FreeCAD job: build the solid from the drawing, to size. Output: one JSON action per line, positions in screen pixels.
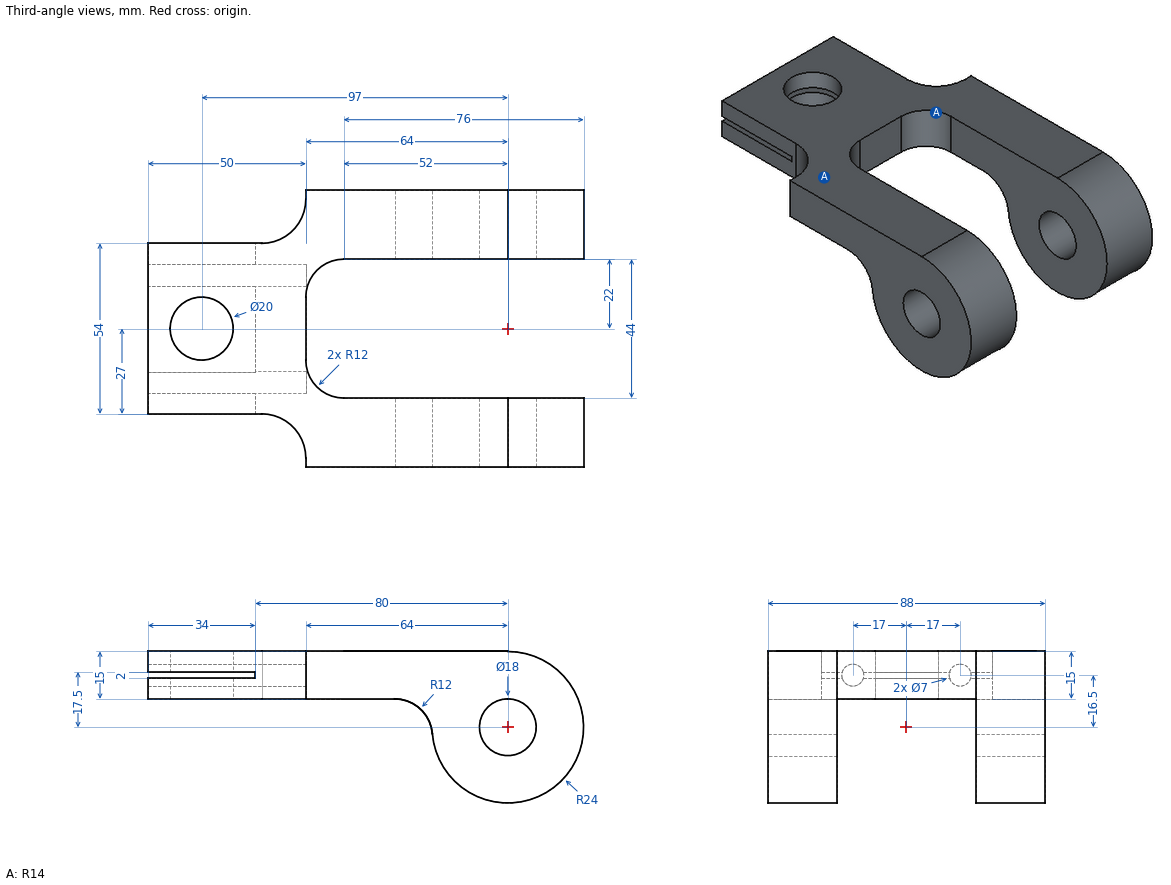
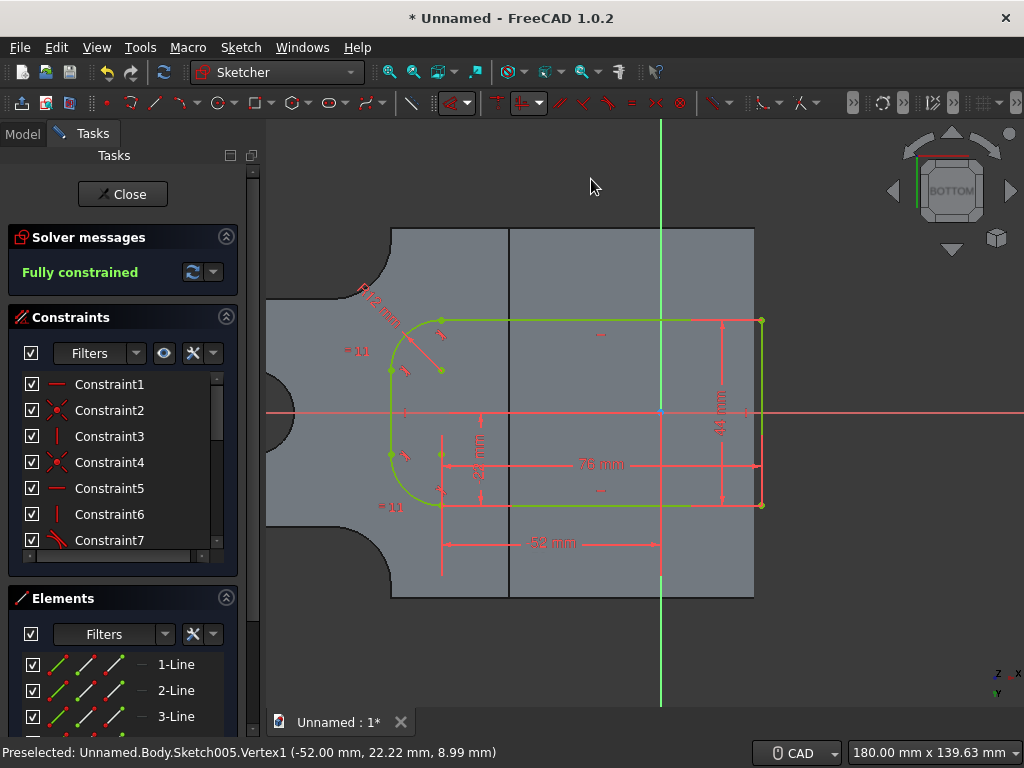
{"action": "left_click", "coordinate": [123, 194]}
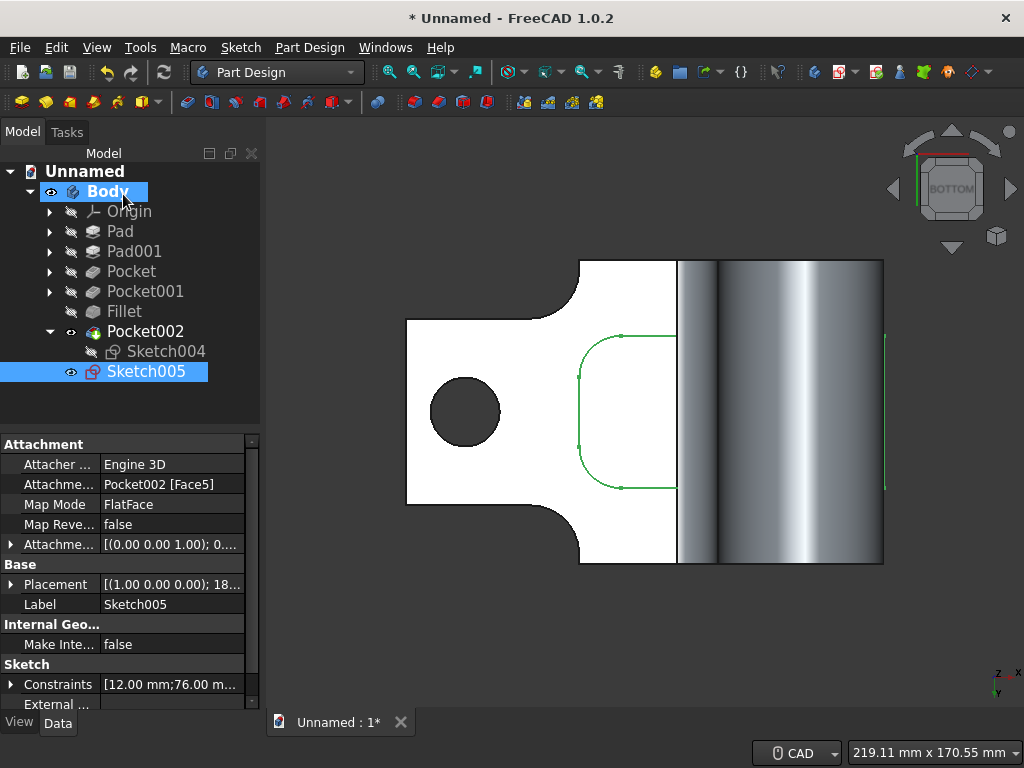
{"action": "left_click", "coordinate": [188, 102]}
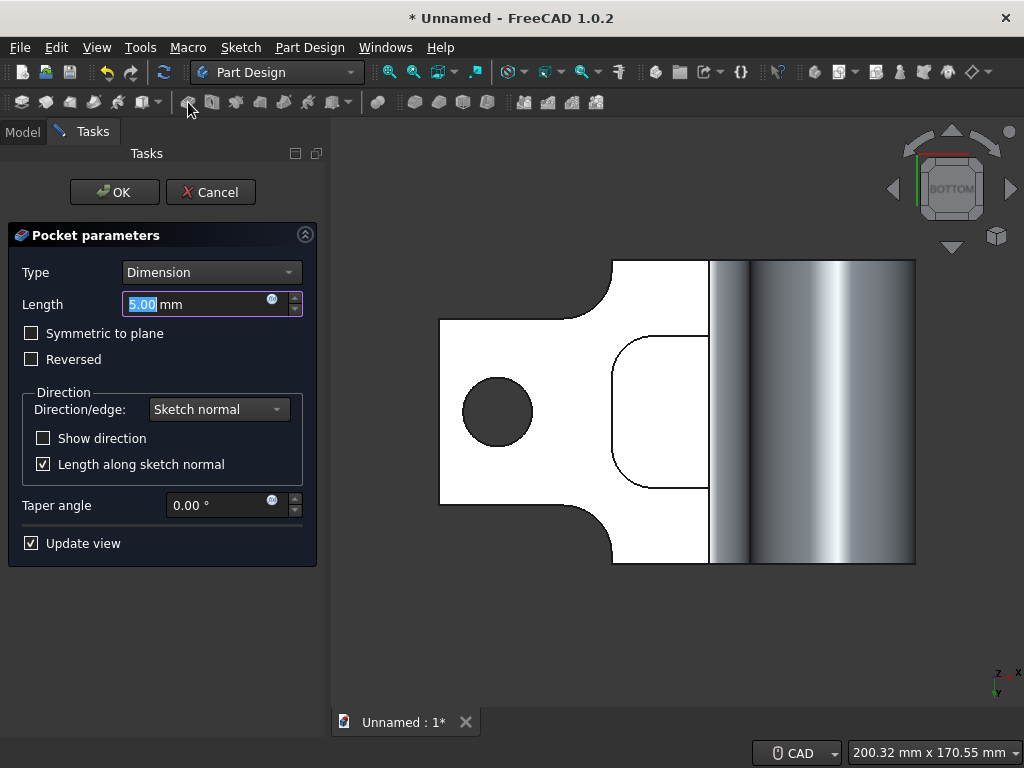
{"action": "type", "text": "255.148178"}
{"action": "key", "text": "Tab"}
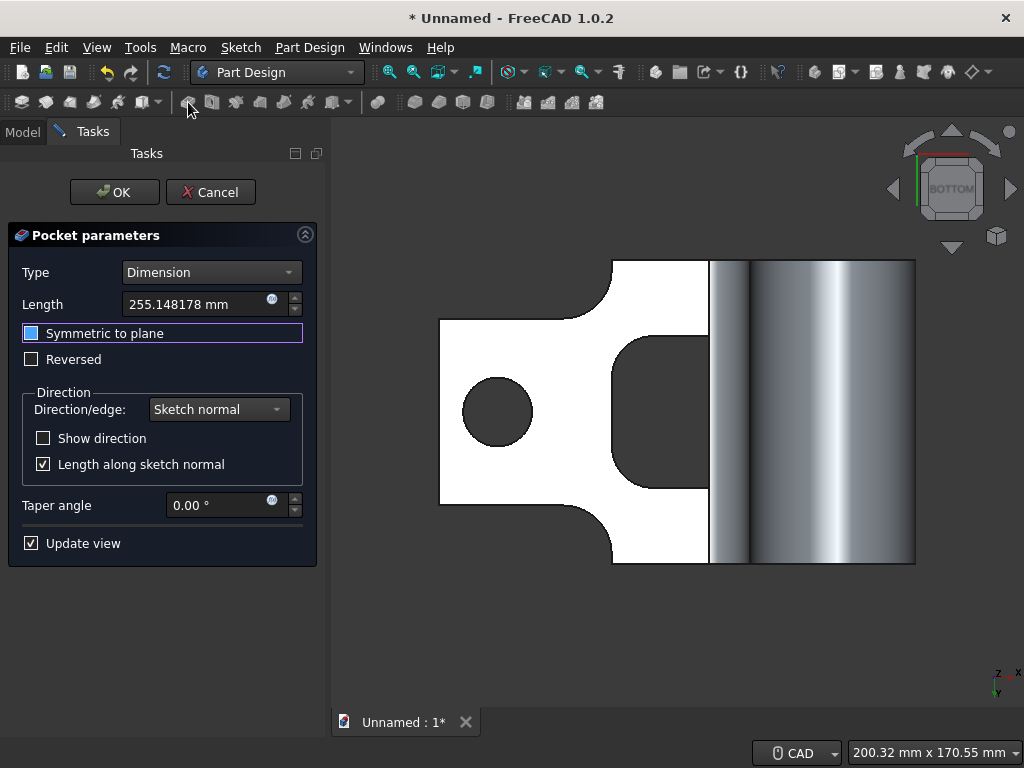
{"action": "left_click", "coordinate": [30, 333]}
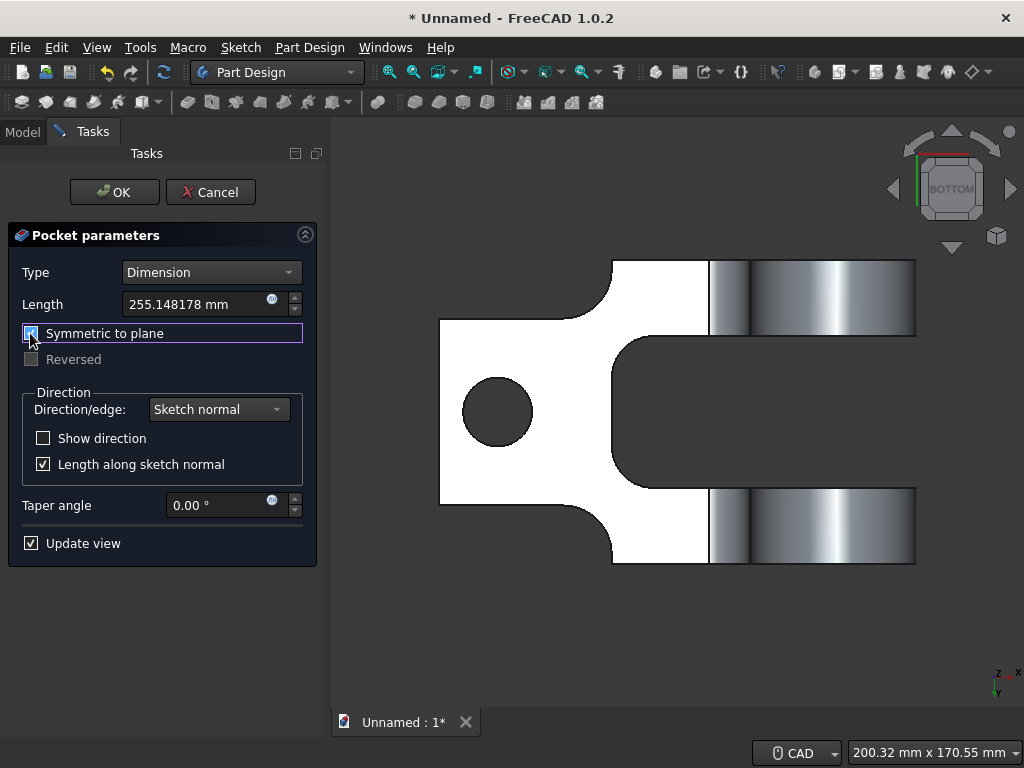
{"action": "left_click", "coordinate": [115, 192]}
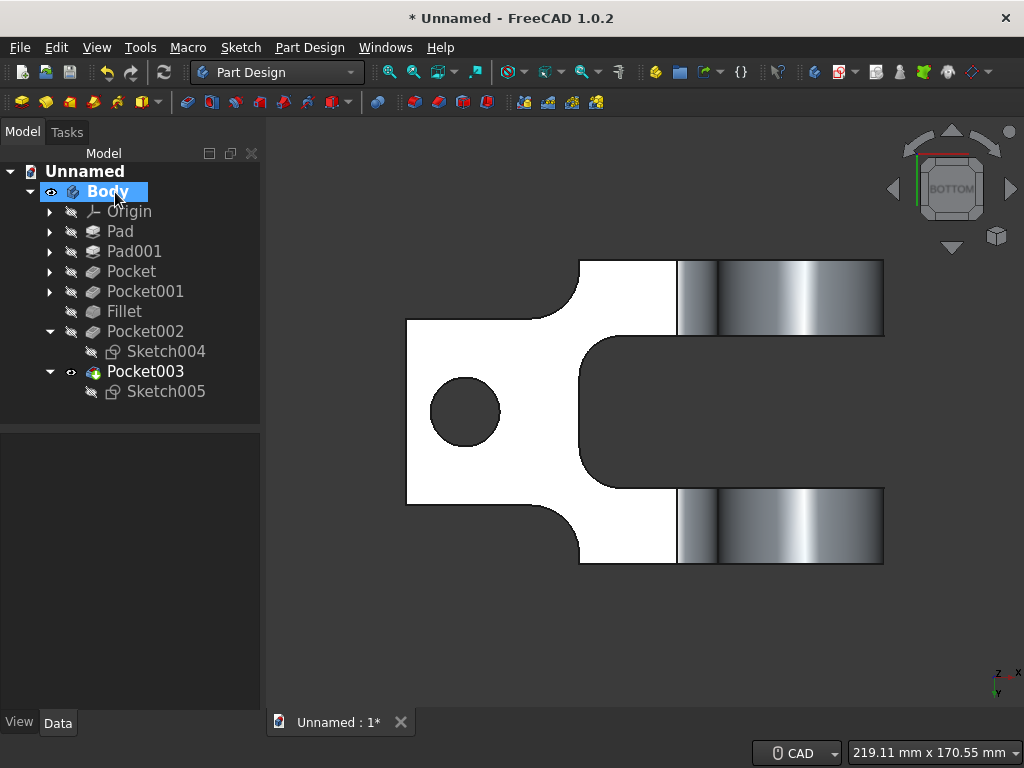
{"action": "key", "text": "0"}